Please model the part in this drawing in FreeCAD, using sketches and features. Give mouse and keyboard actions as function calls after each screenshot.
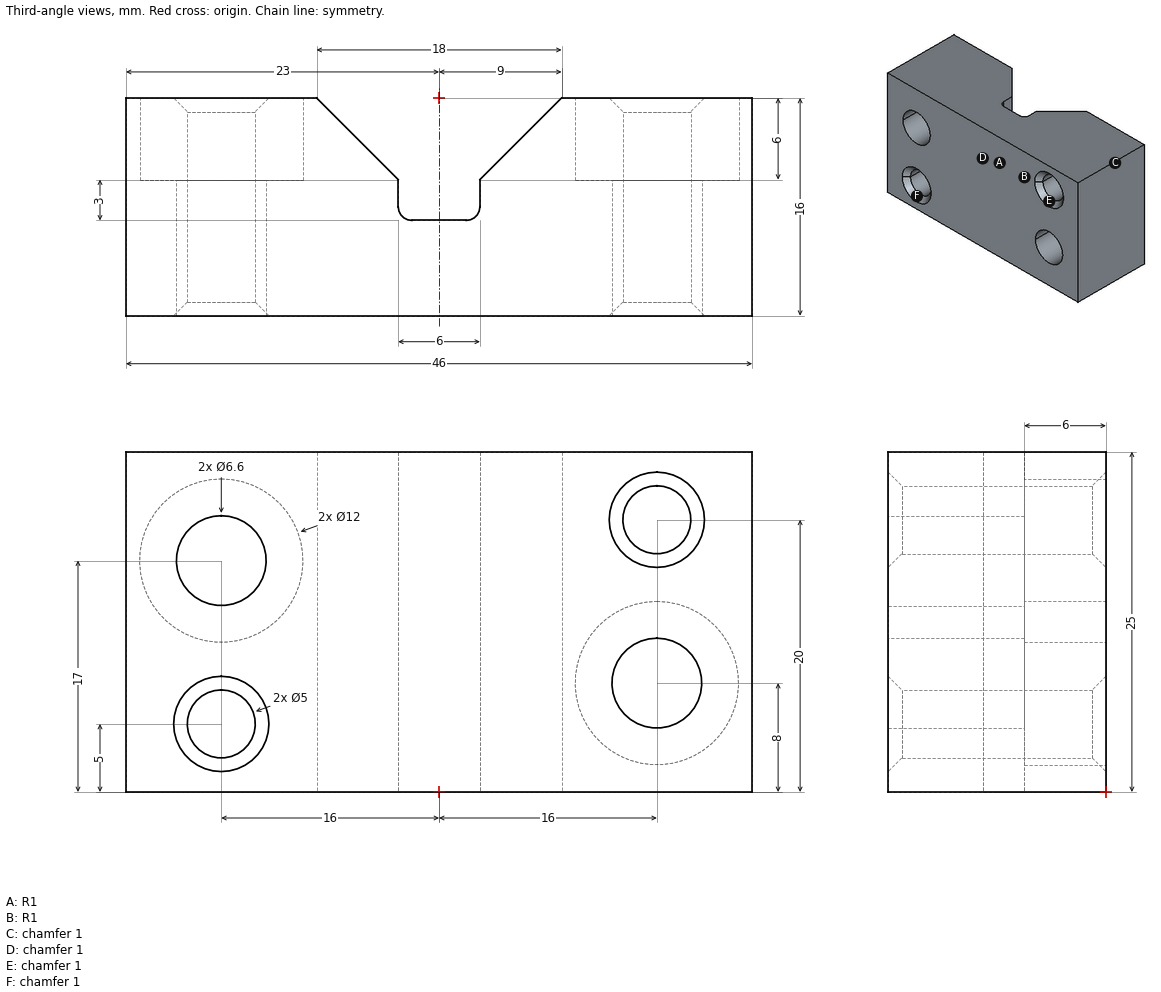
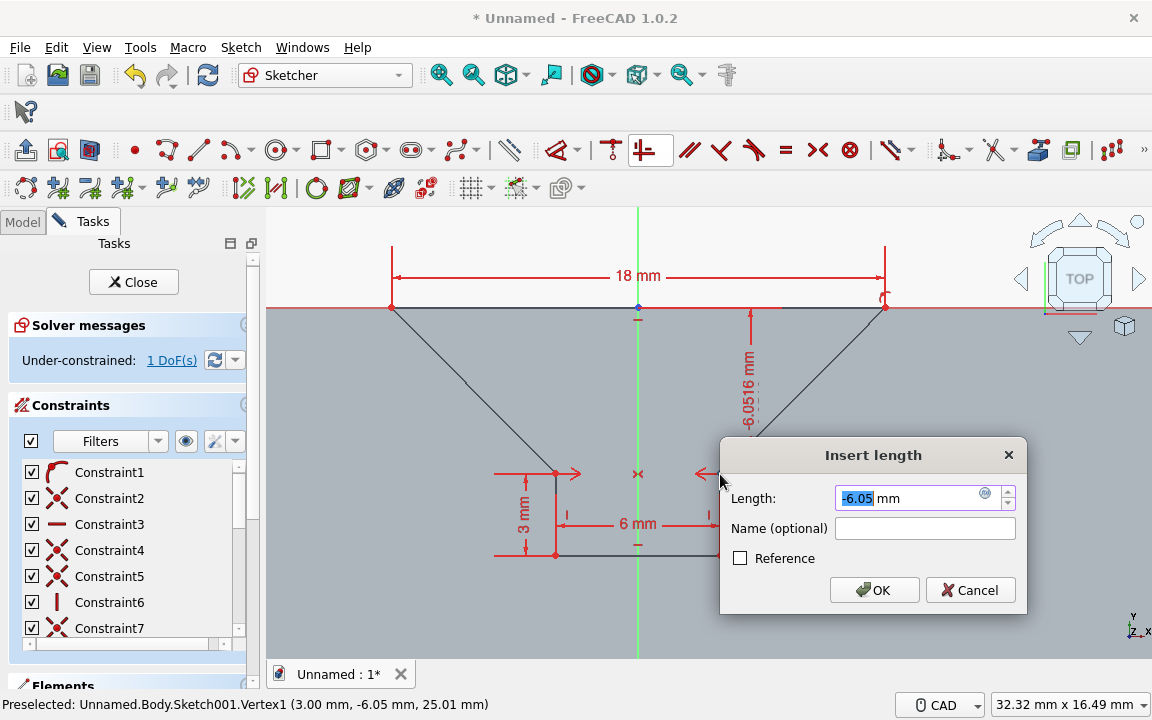
text(-6)
key(Return)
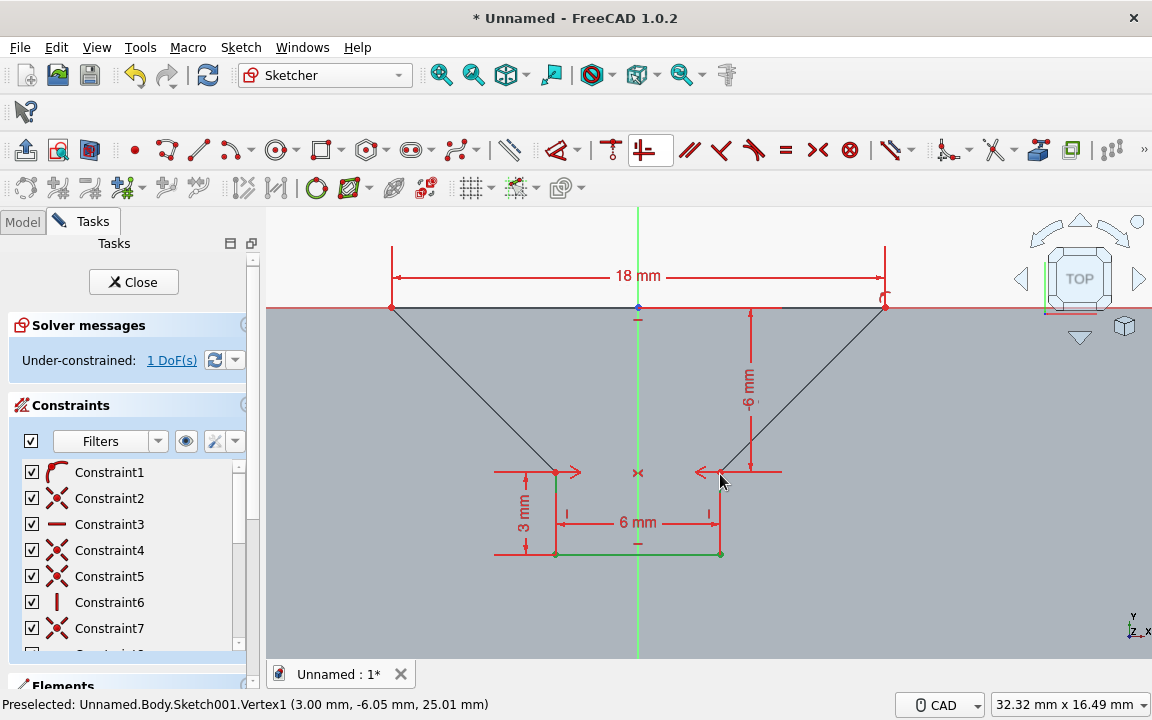
click(885, 308)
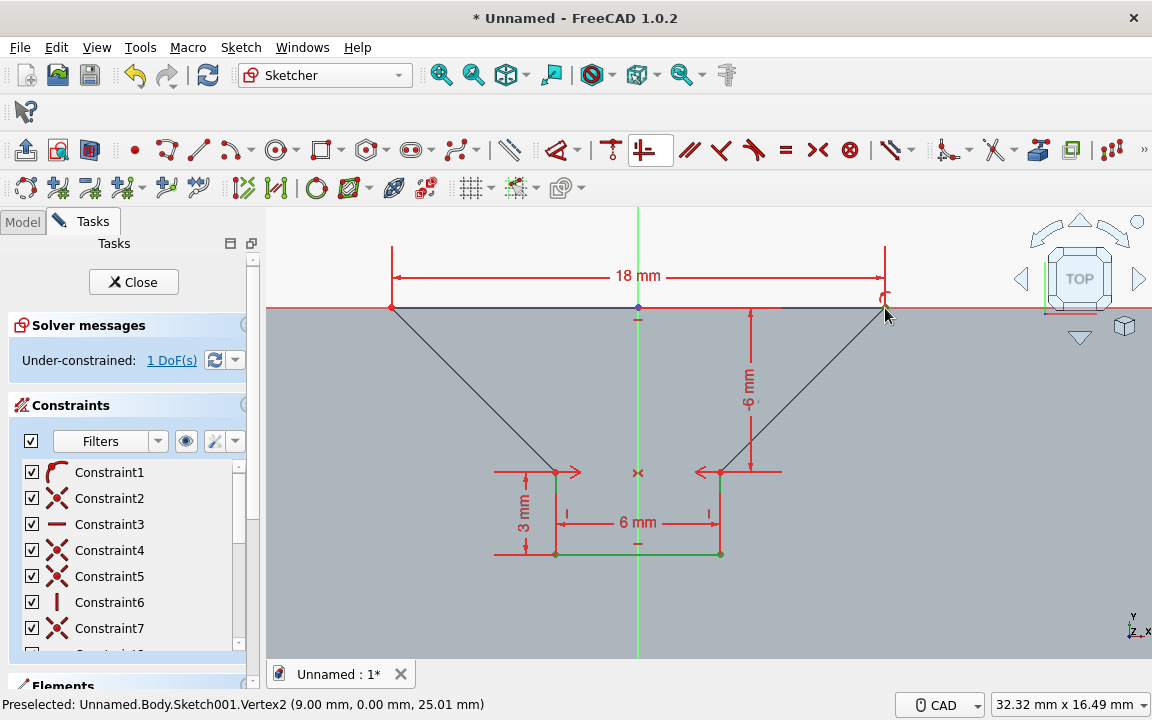
key(l)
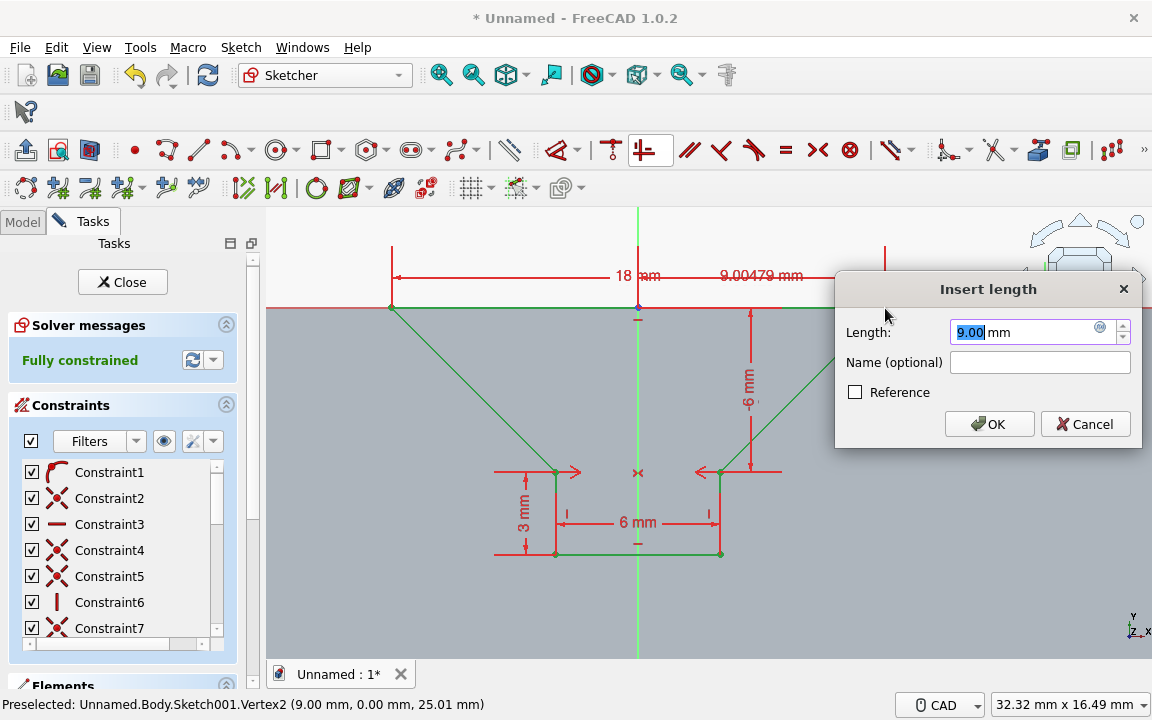
text(9)
key(Return)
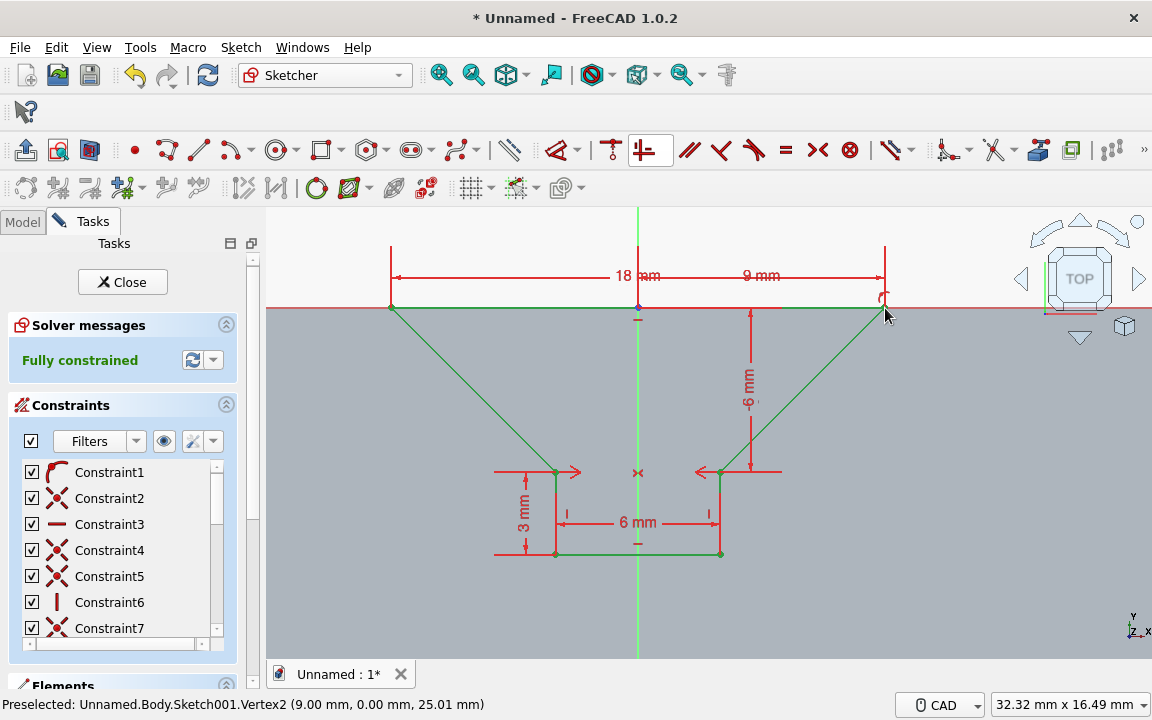
click(123, 282)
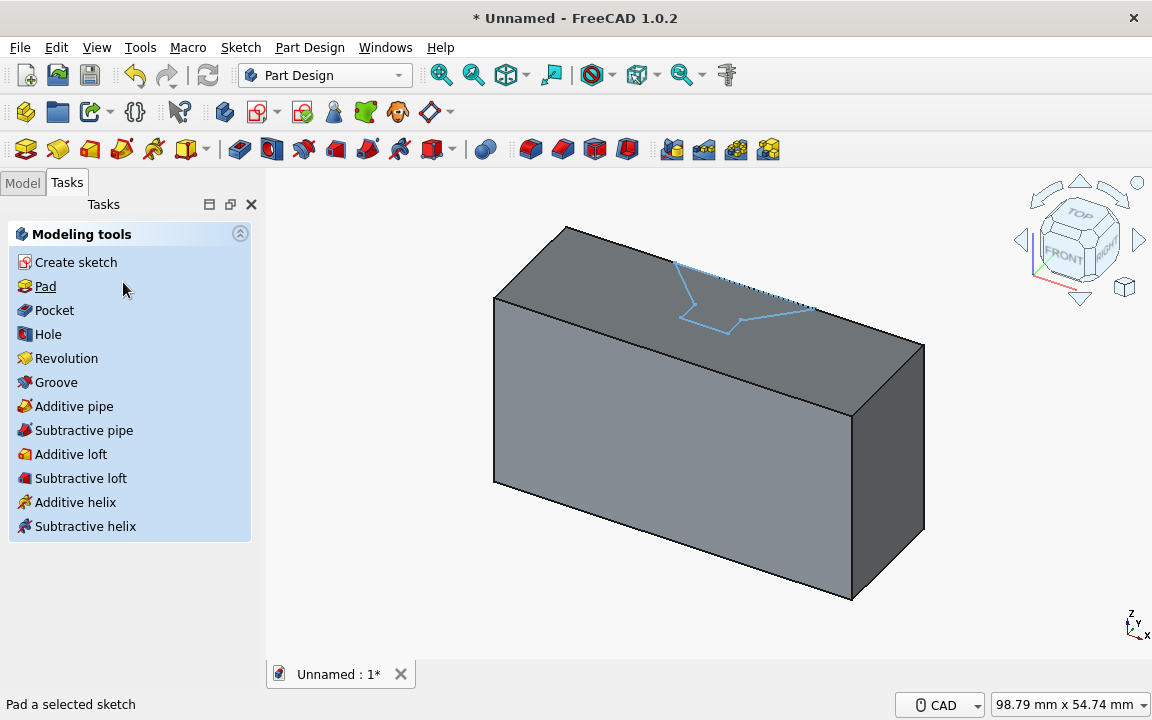
click(240, 150)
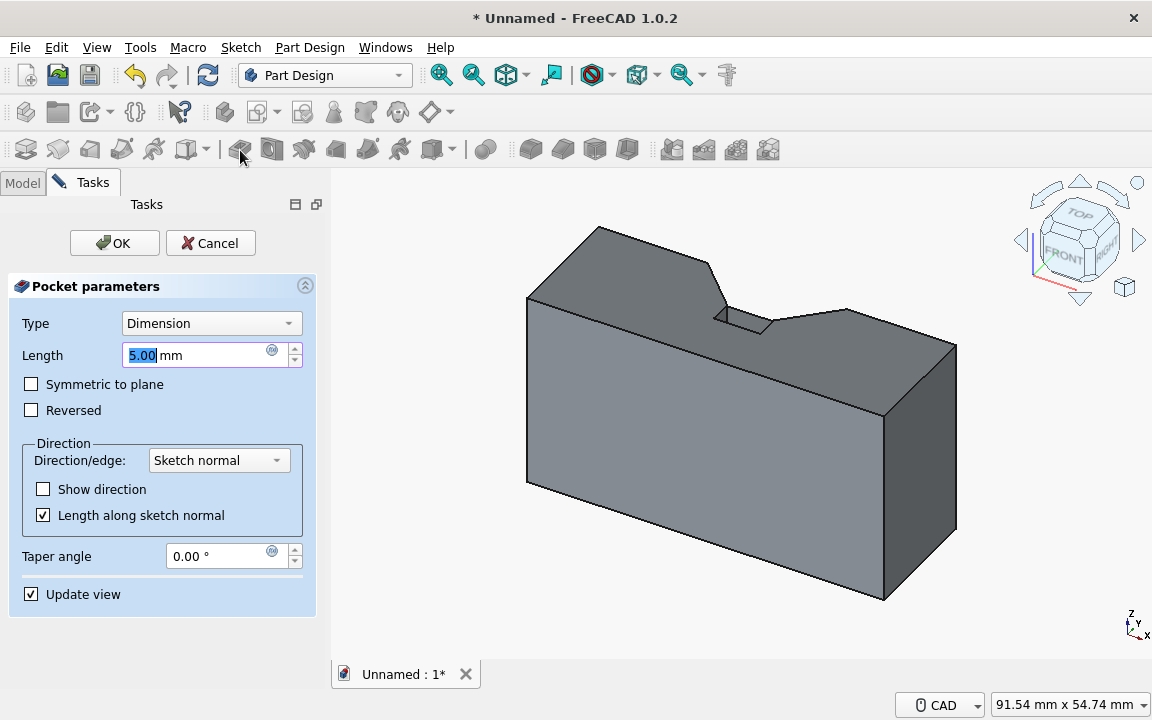
click(212, 324)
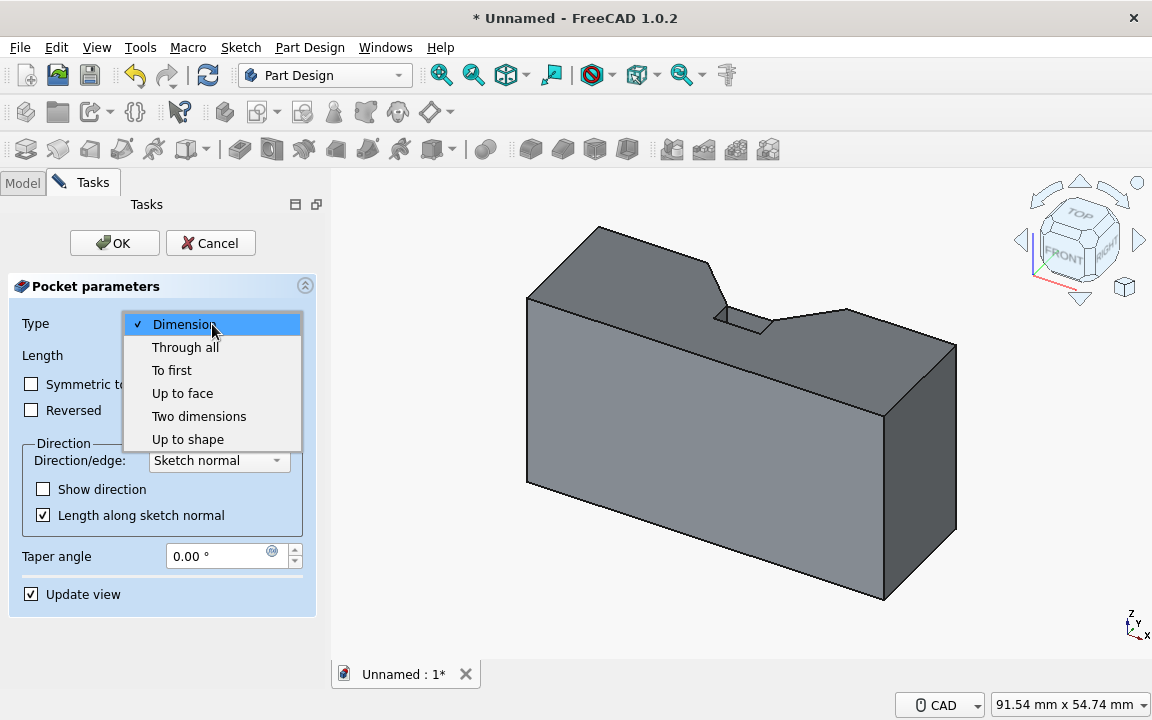
click(212, 348)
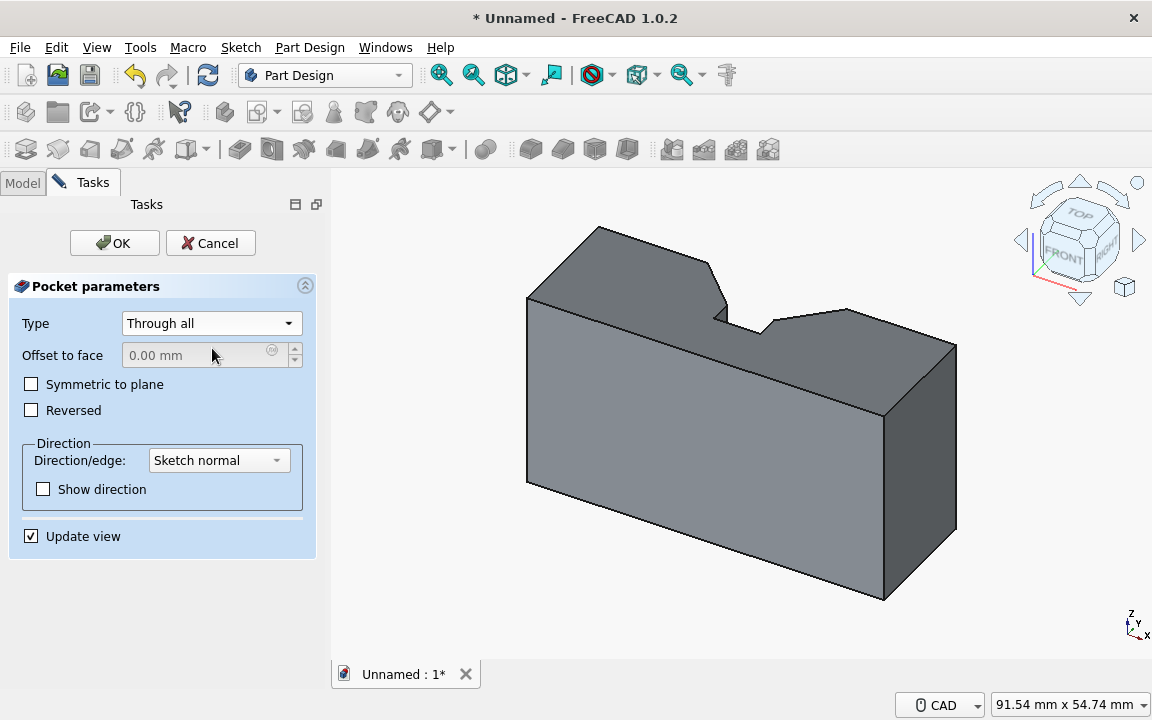
click(115, 243)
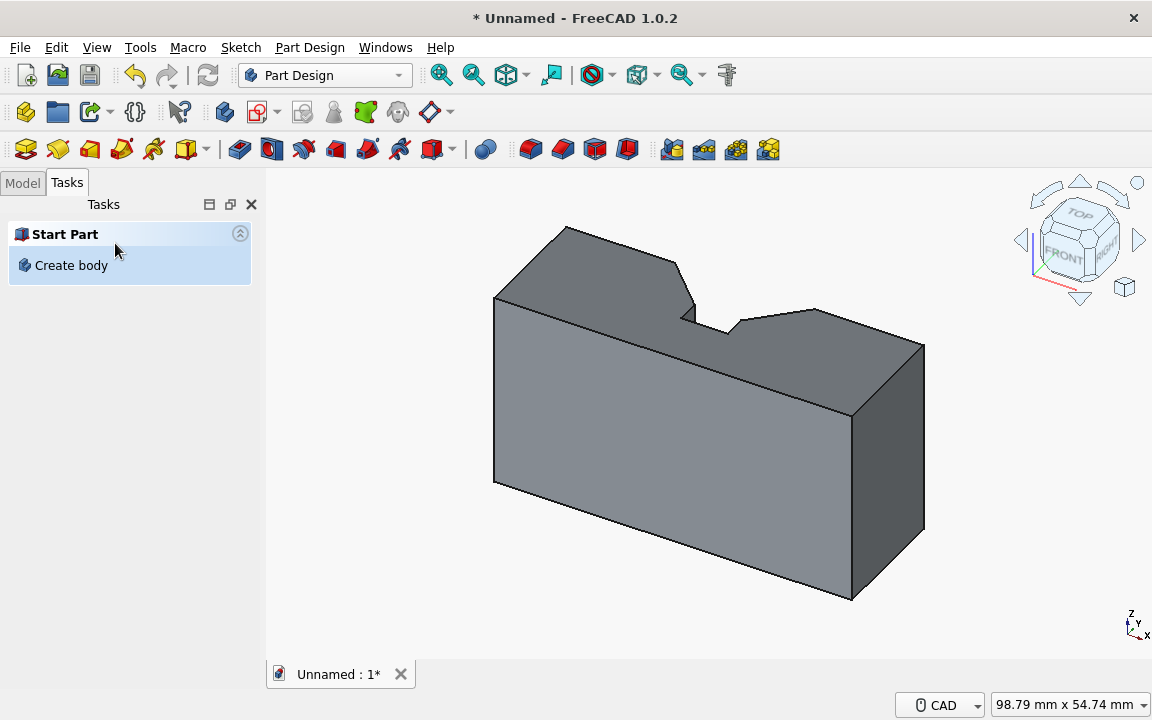
key(4)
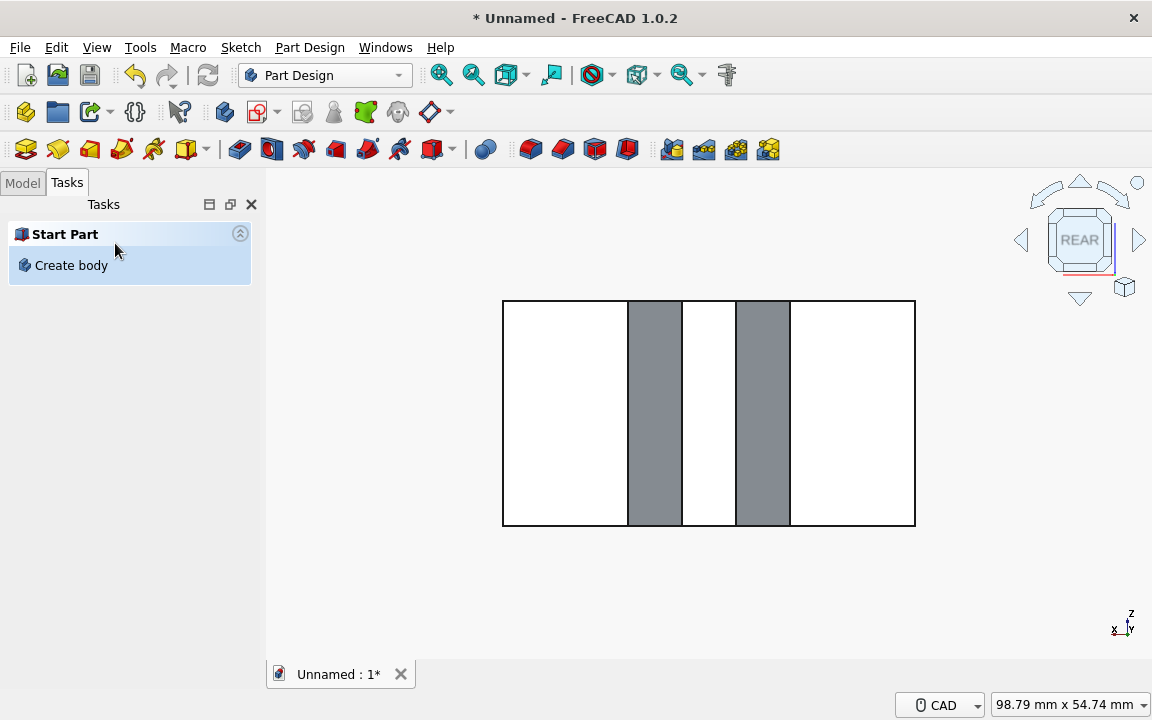
click(853, 380)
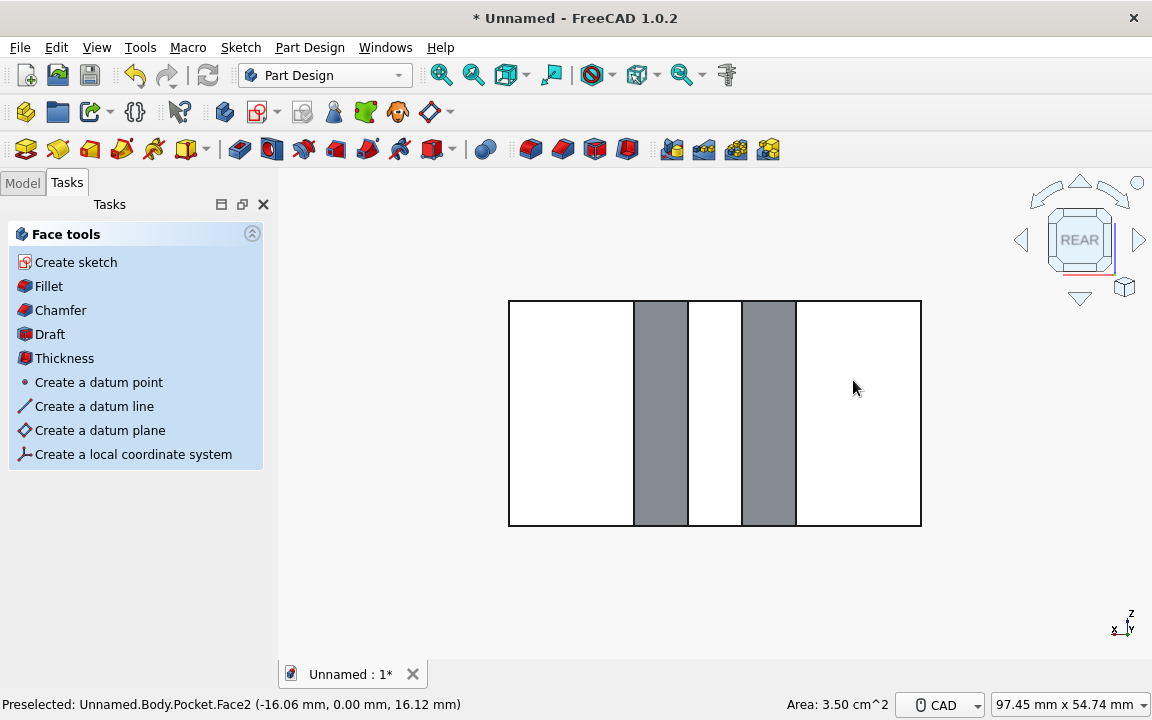
click(258, 112)